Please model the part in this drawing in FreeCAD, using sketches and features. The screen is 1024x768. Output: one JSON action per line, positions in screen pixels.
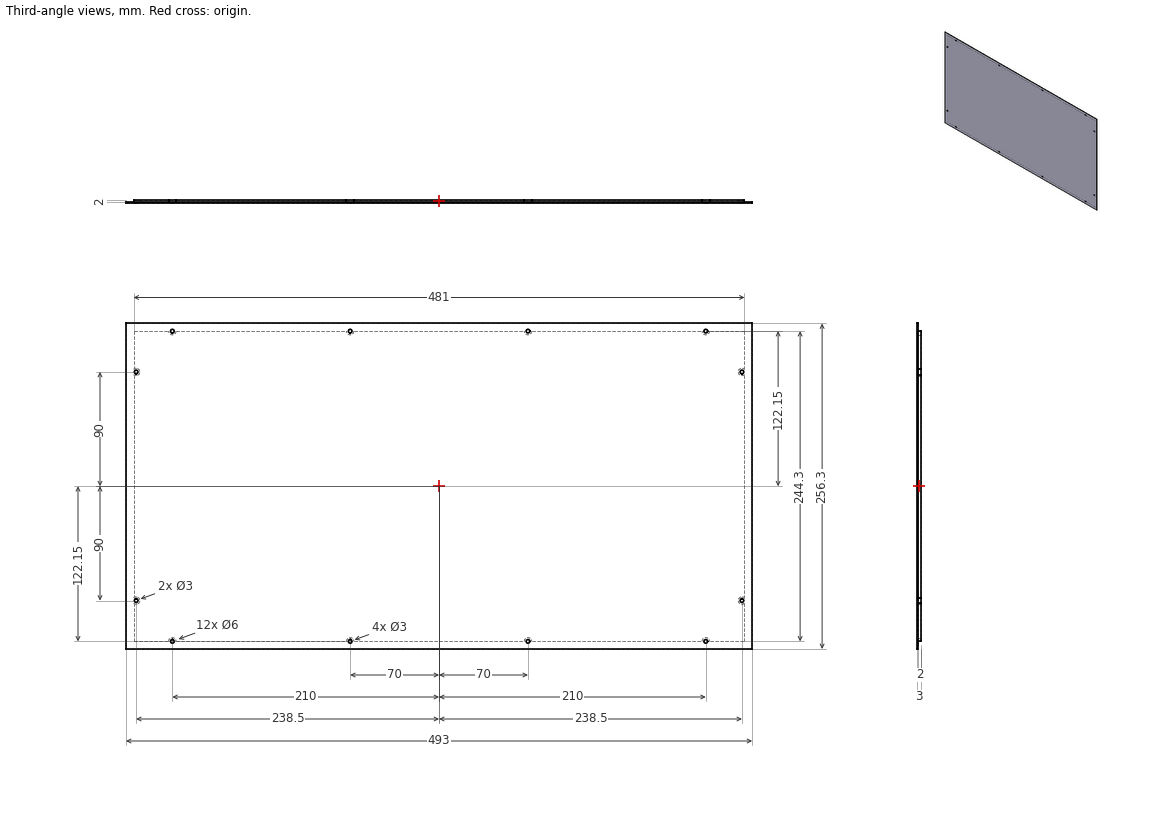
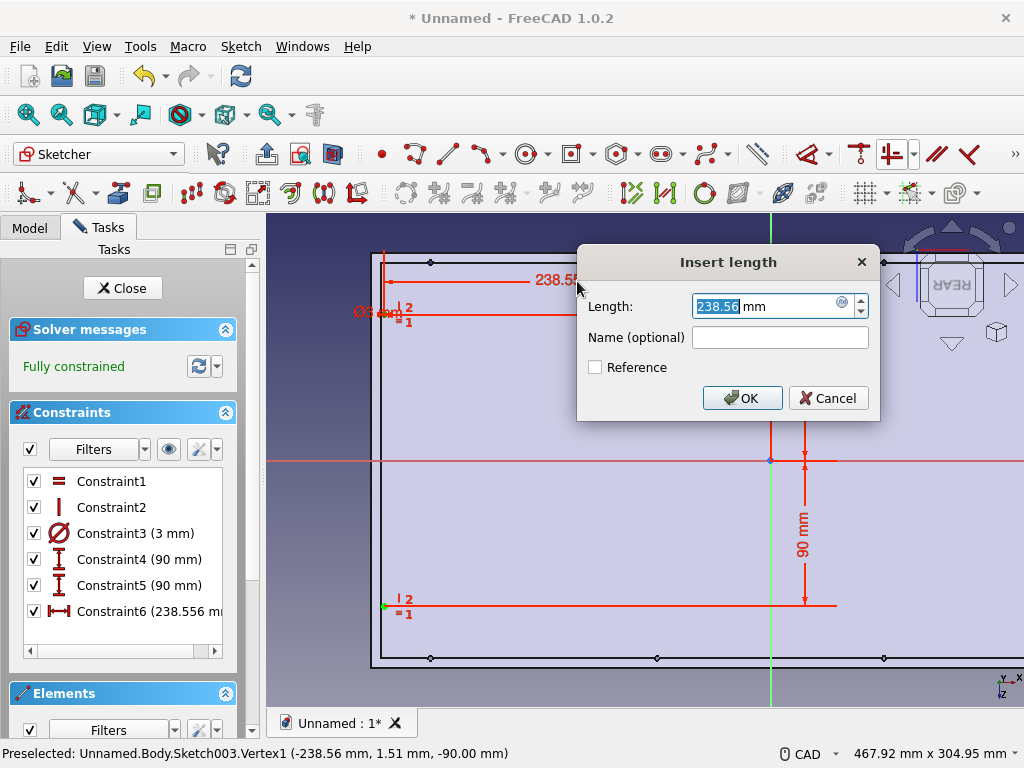
{"action": "type", "text": "238.5"}
{"action": "key", "text": "Return"}
{"action": "key", "text": "Escape"}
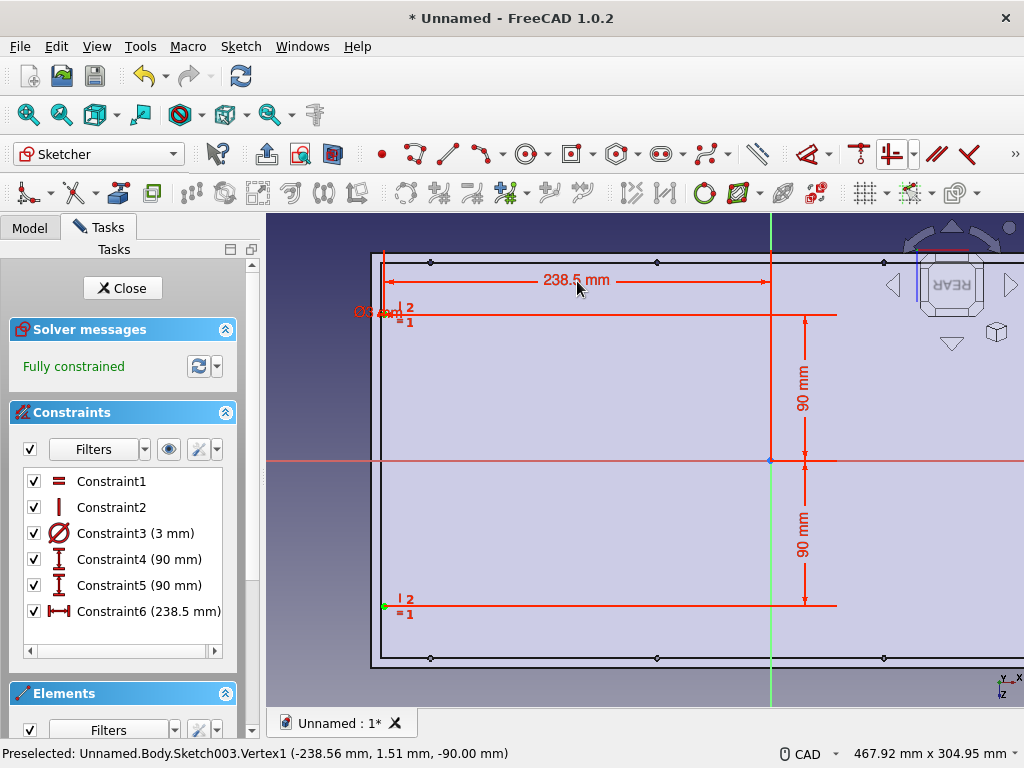
{"action": "left_click", "coordinate": [123, 288]}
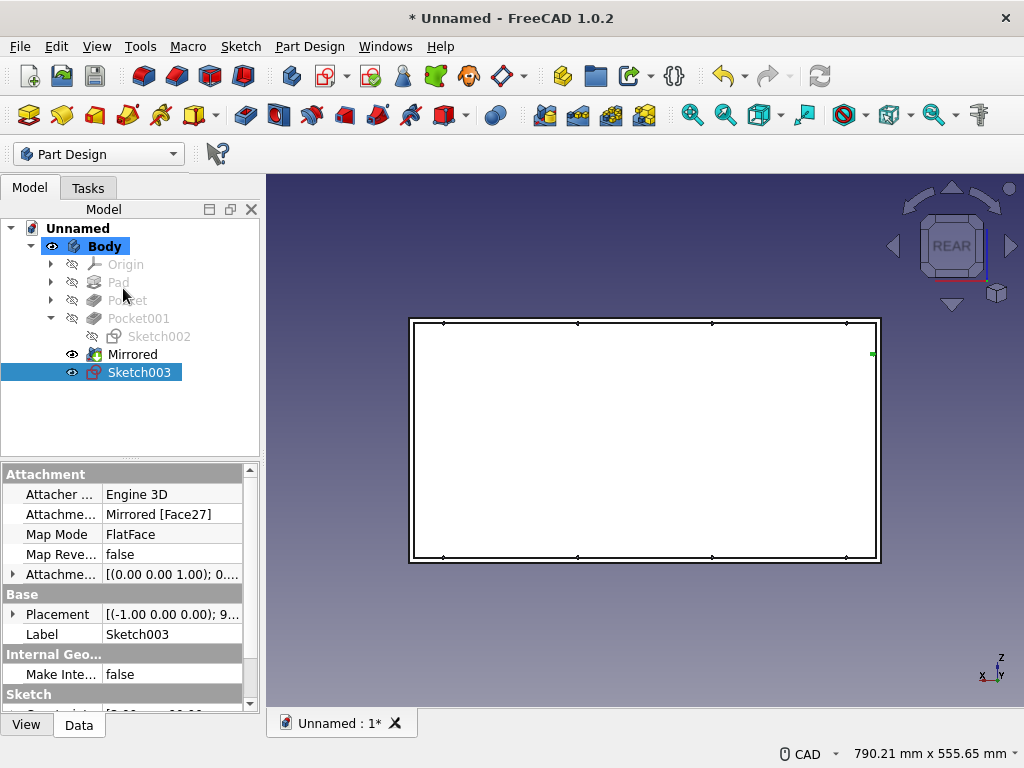
{"action": "left_click", "coordinate": [246, 116]}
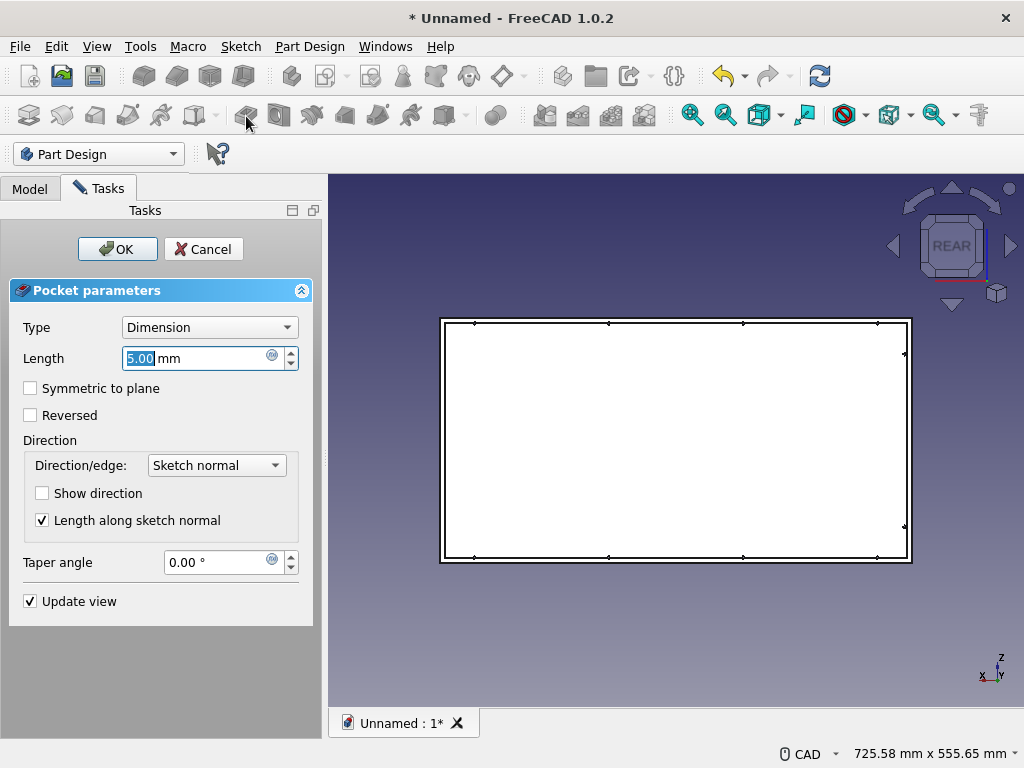
{"action": "left_click", "coordinate": [210, 328]}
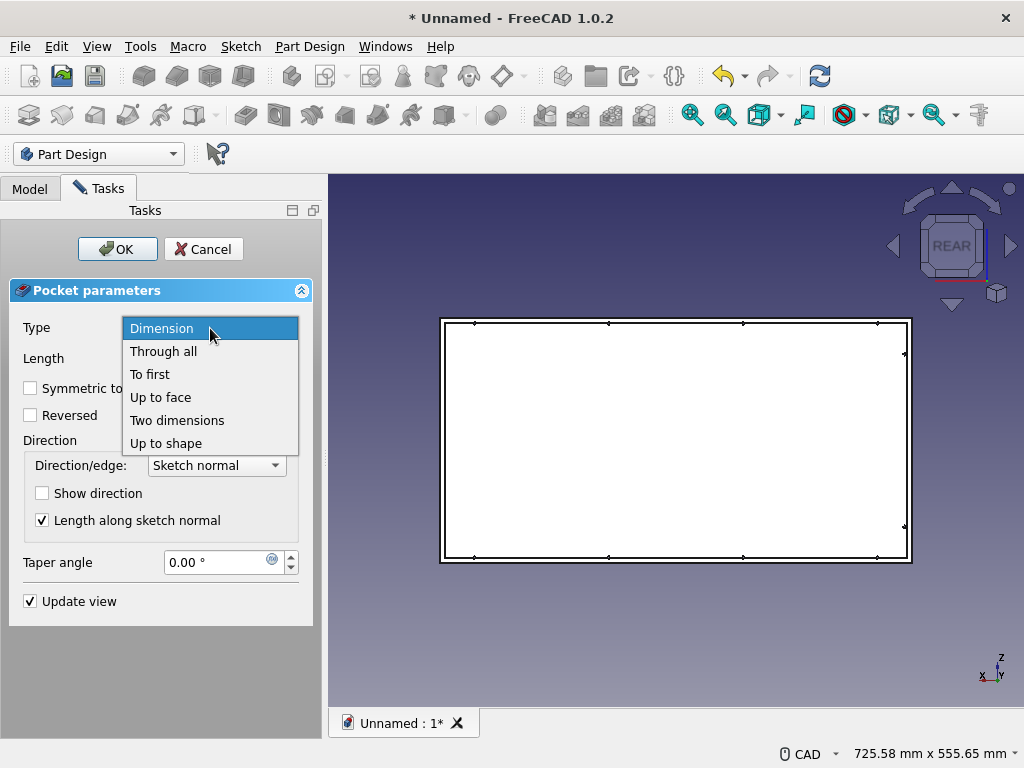
{"action": "left_click", "coordinate": [208, 352]}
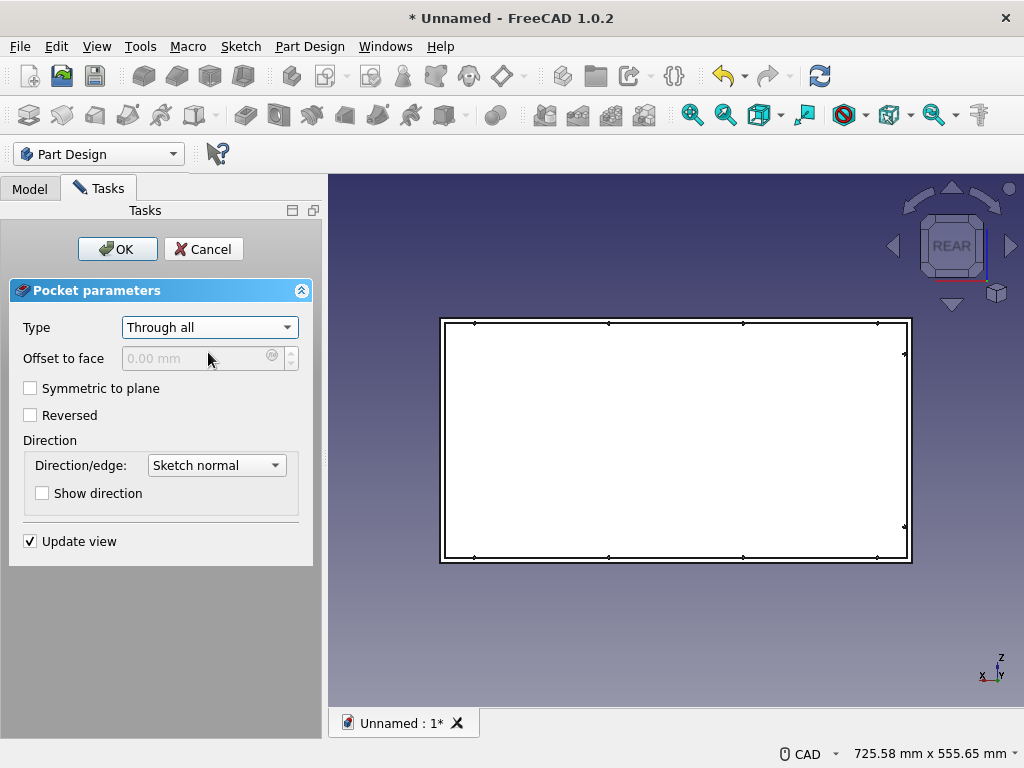
{"action": "left_click", "coordinate": [118, 249]}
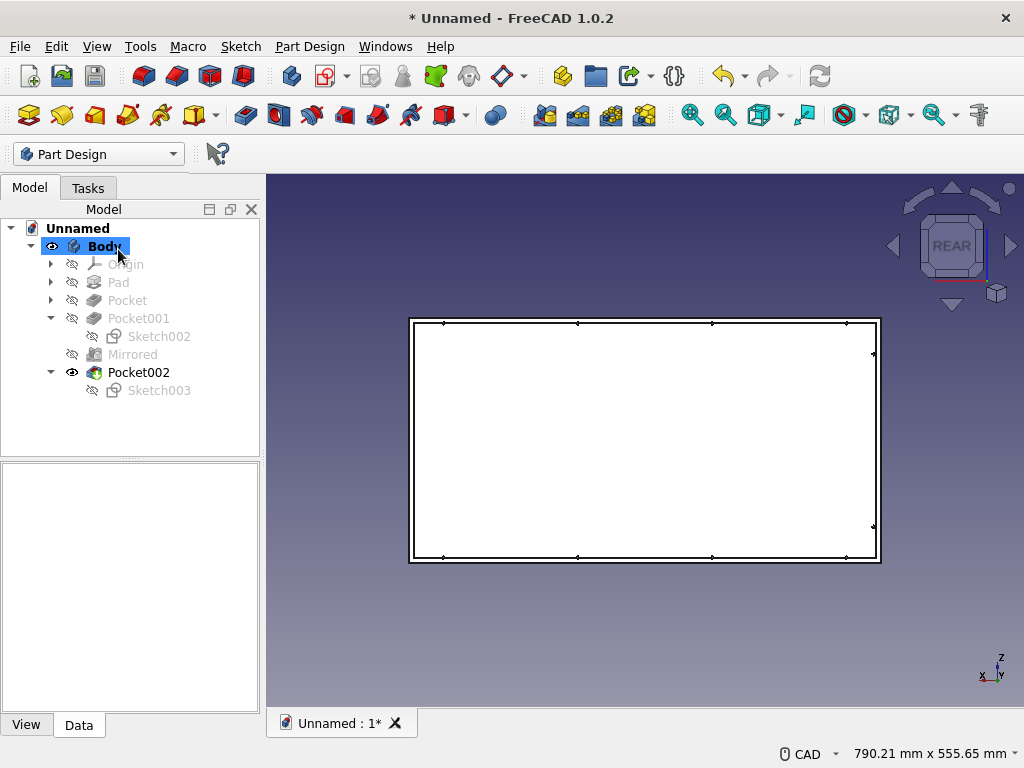
{"action": "left_click", "coordinate": [117, 372]}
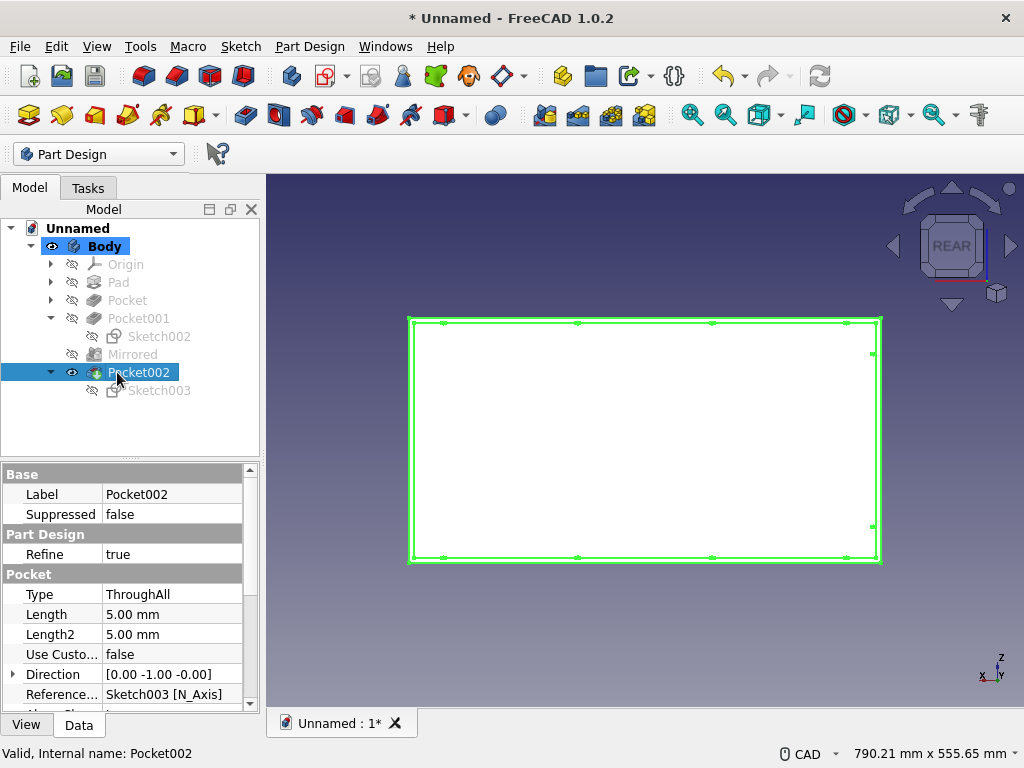
{"action": "left_click", "coordinate": [545, 116]}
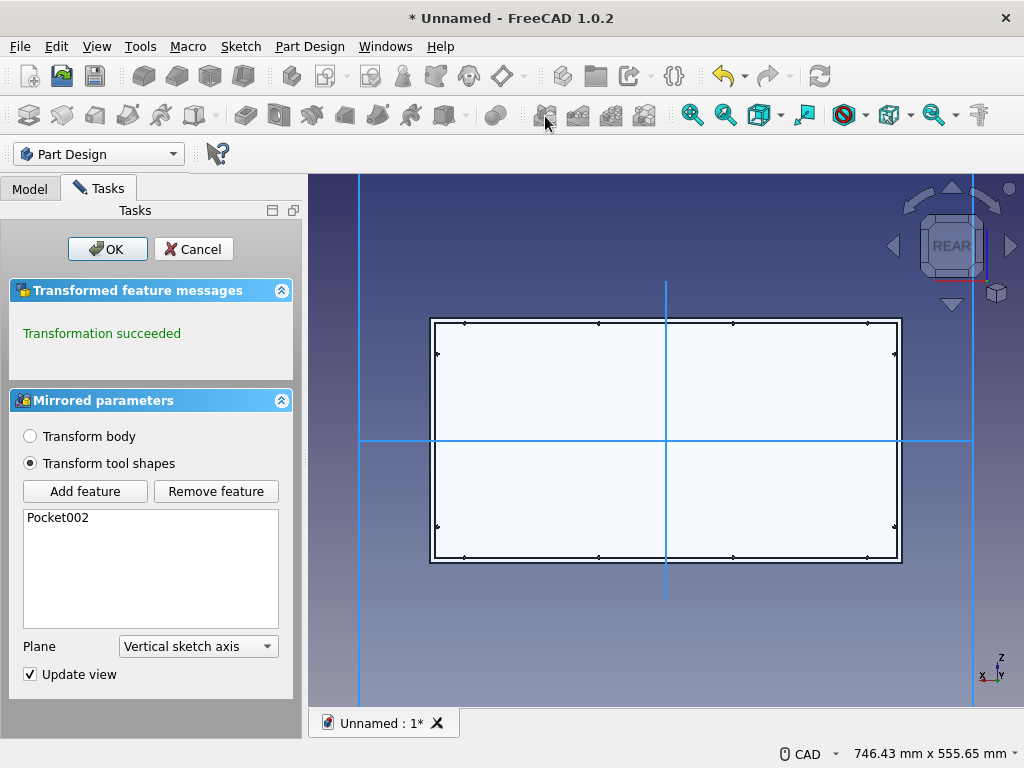
{"action": "left_click", "coordinate": [199, 646]}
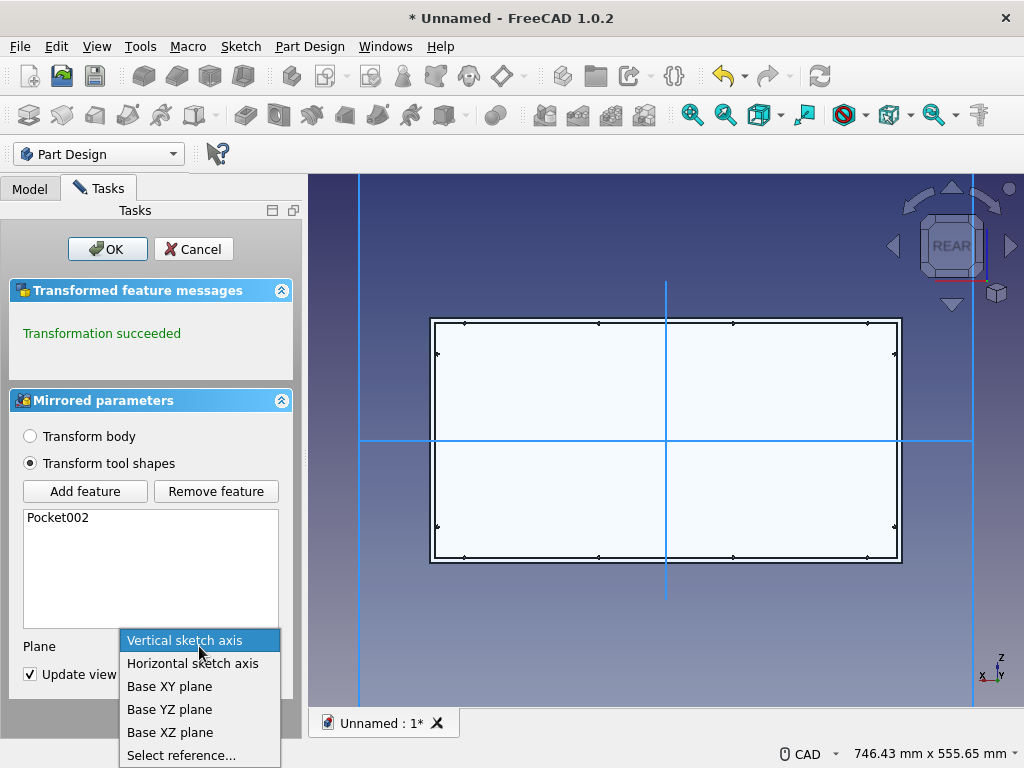
{"action": "left_click", "coordinate": [198, 710]}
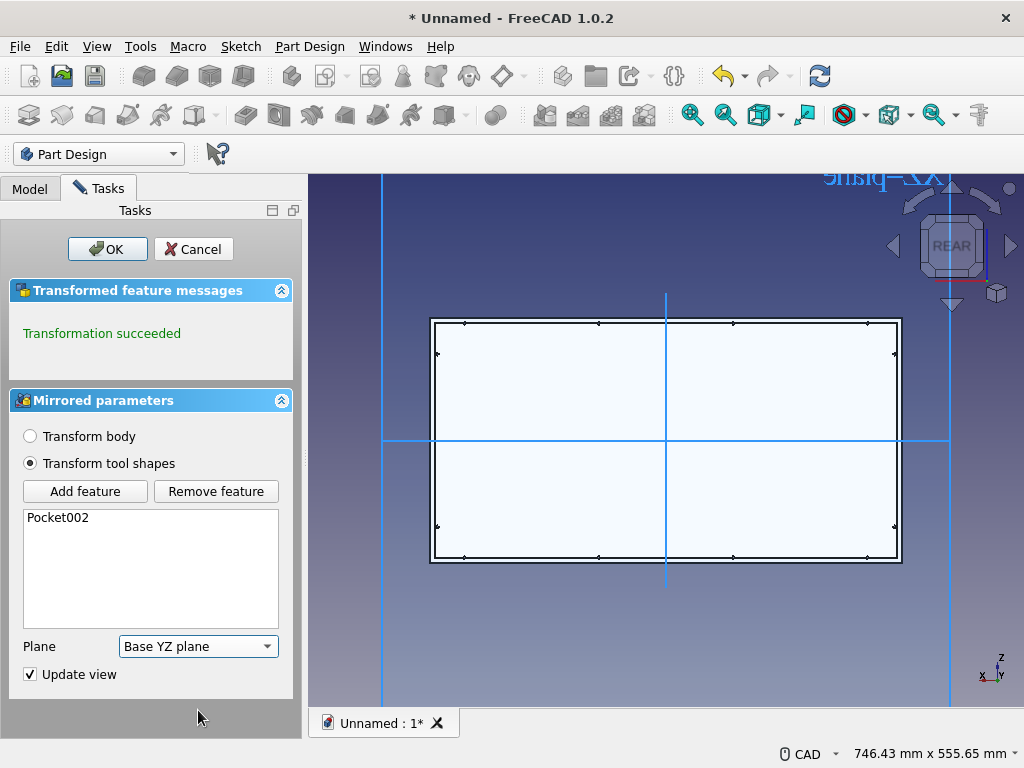
{"action": "left_click", "coordinate": [108, 249]}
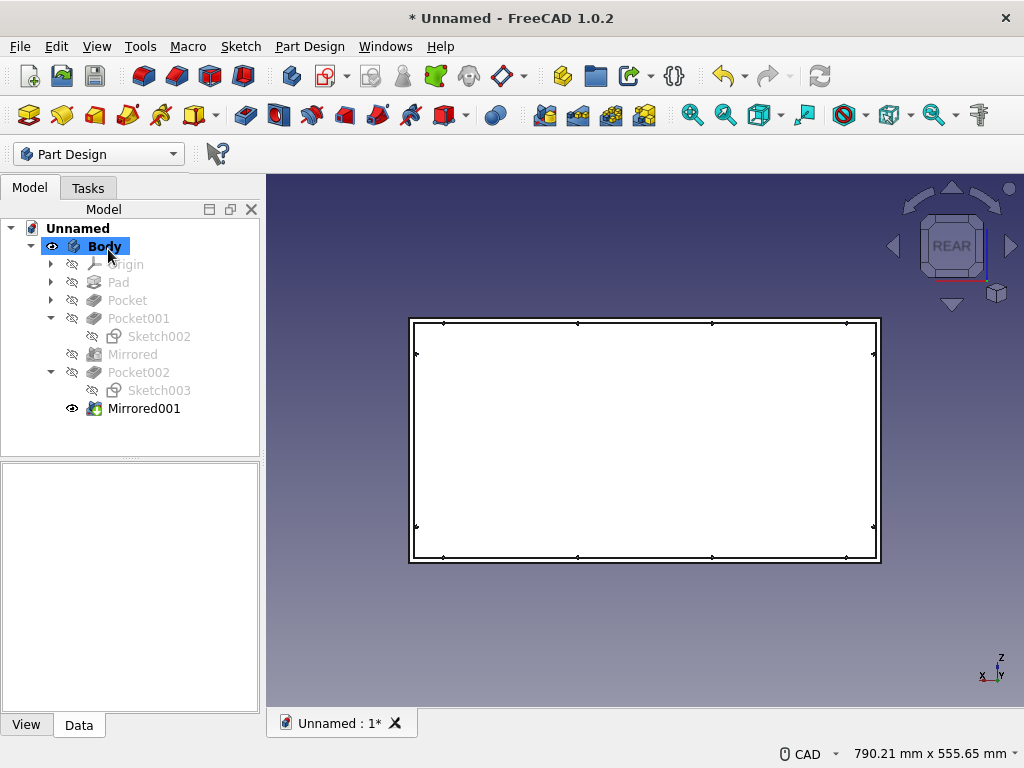
{"action": "left_click", "coordinate": [645, 440]}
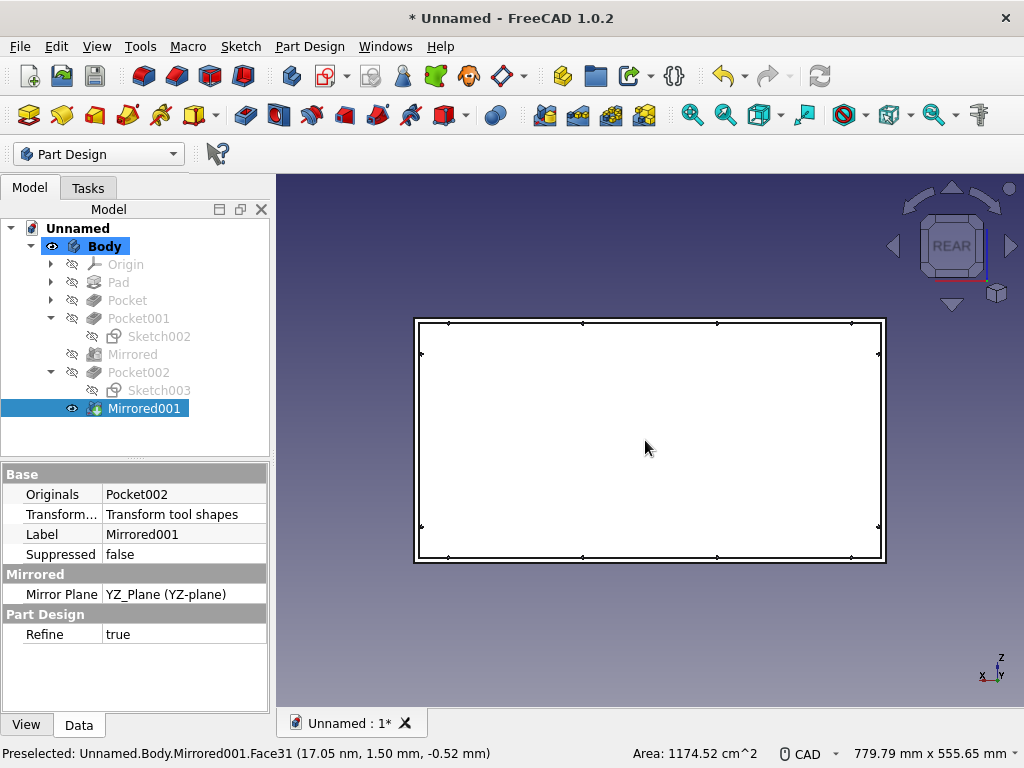
{"action": "left_click", "coordinate": [324, 76]}